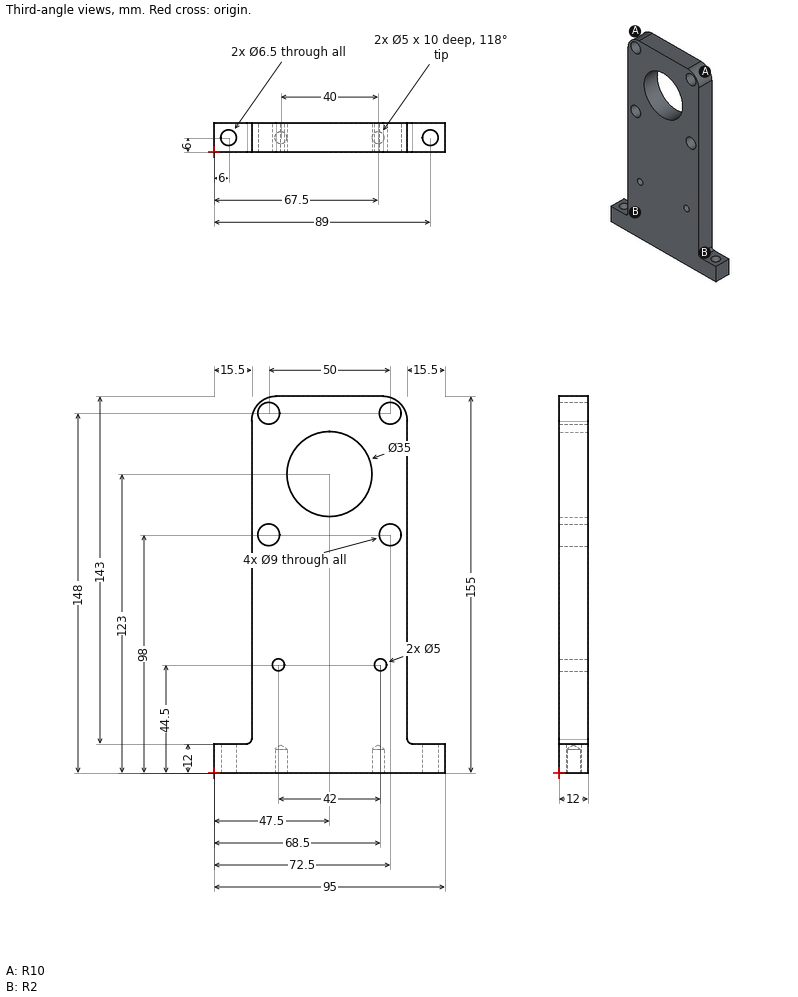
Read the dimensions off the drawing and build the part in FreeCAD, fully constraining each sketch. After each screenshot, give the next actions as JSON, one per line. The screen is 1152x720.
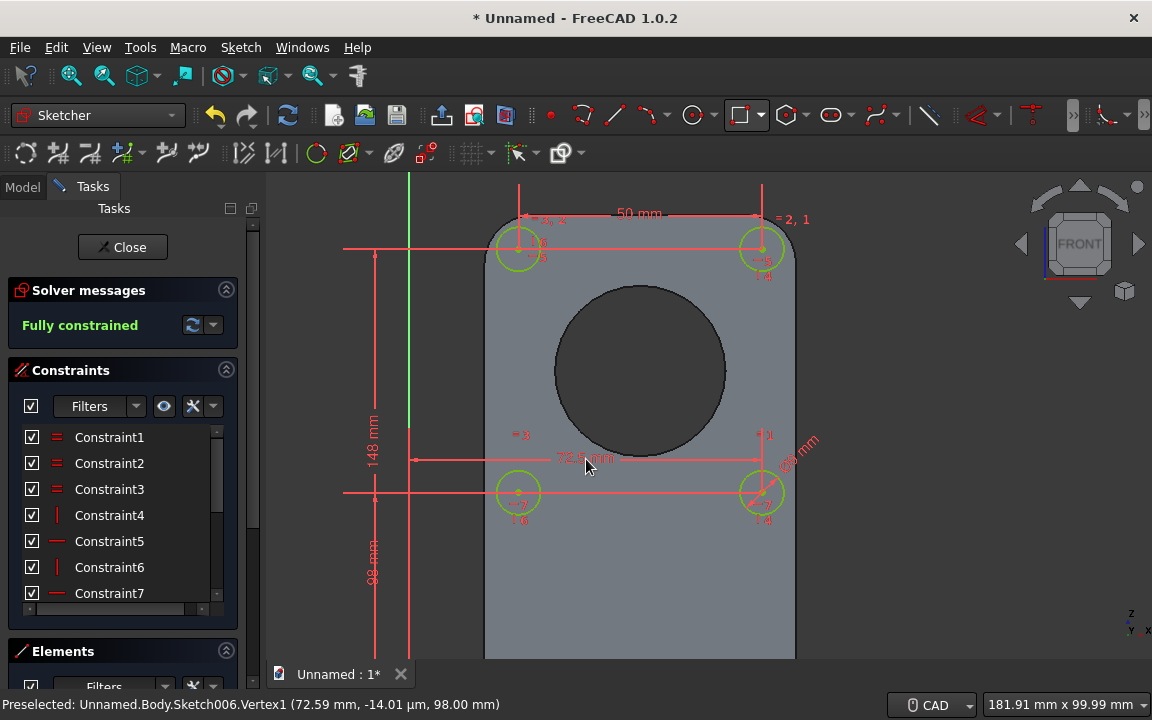
{"action": "left_click", "coordinate": [123, 247]}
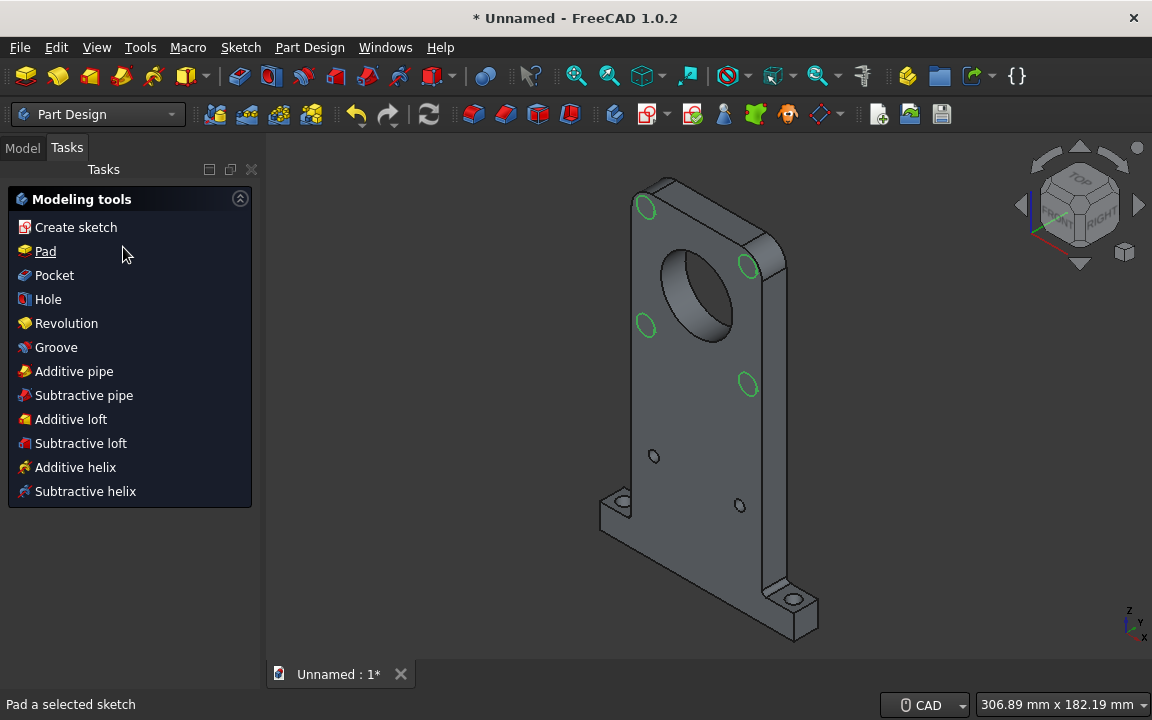
{"action": "left_click", "coordinate": [272, 76]}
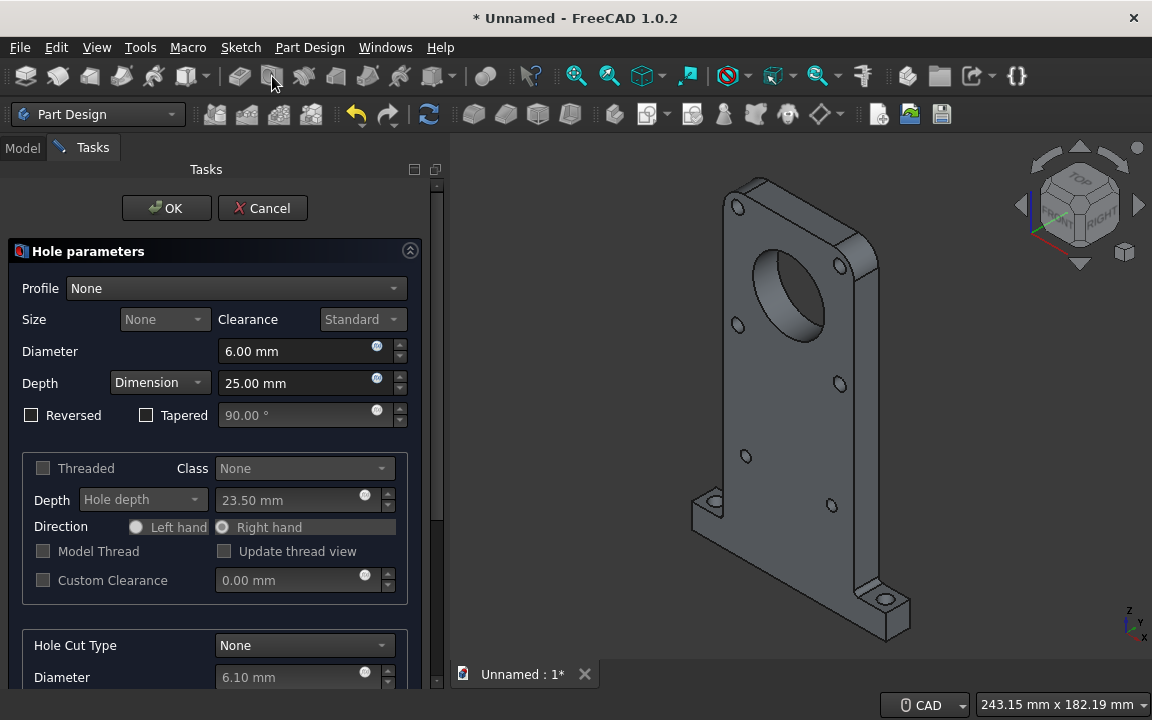
{"action": "triple_click", "coordinate": [305, 351]}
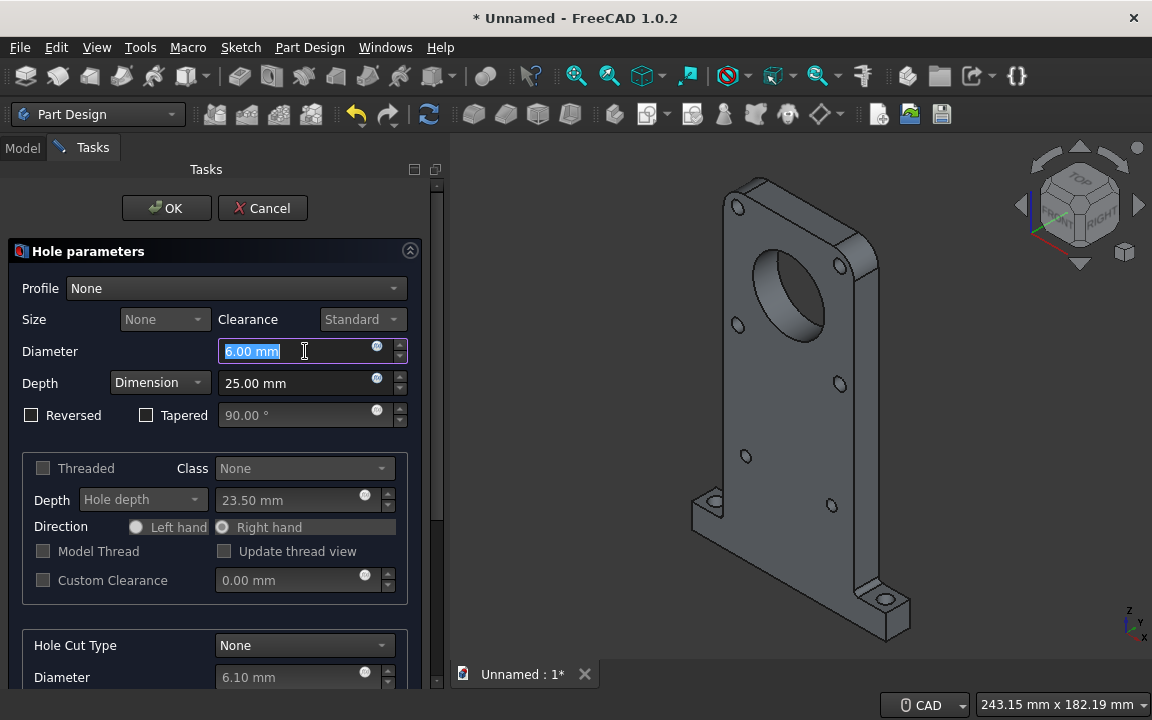
{"action": "type", "text": "9"}
{"action": "key", "text": "Tab"}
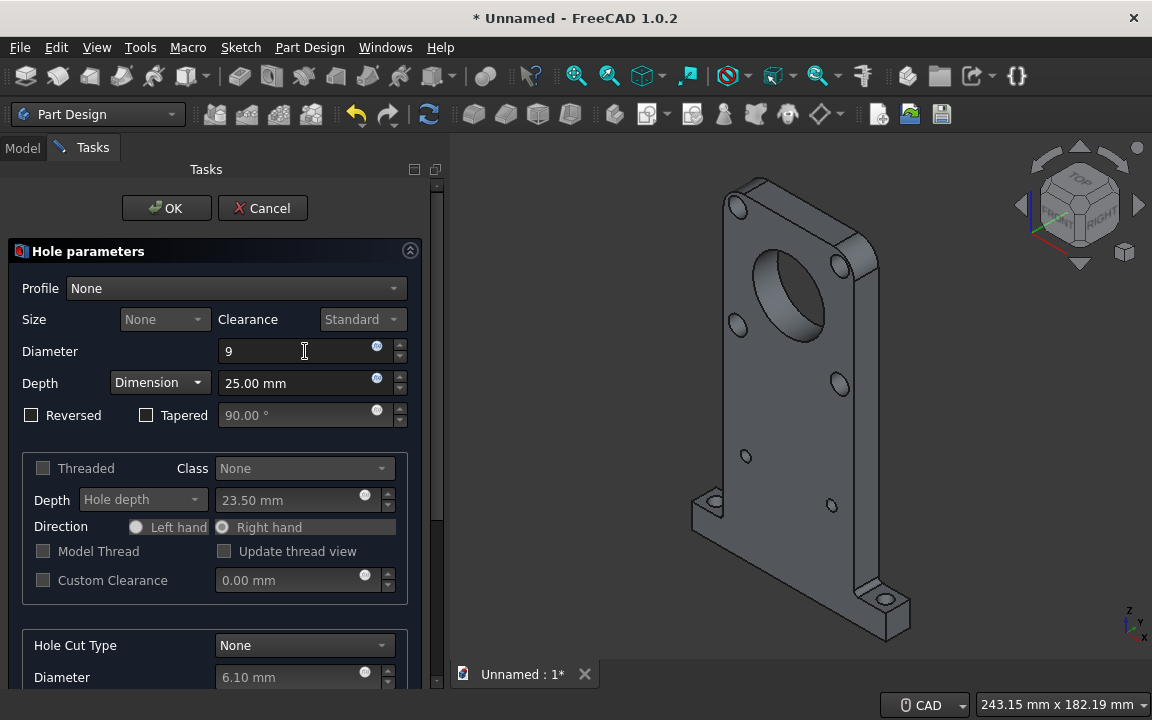
{"action": "left_click", "coordinate": [161, 382]}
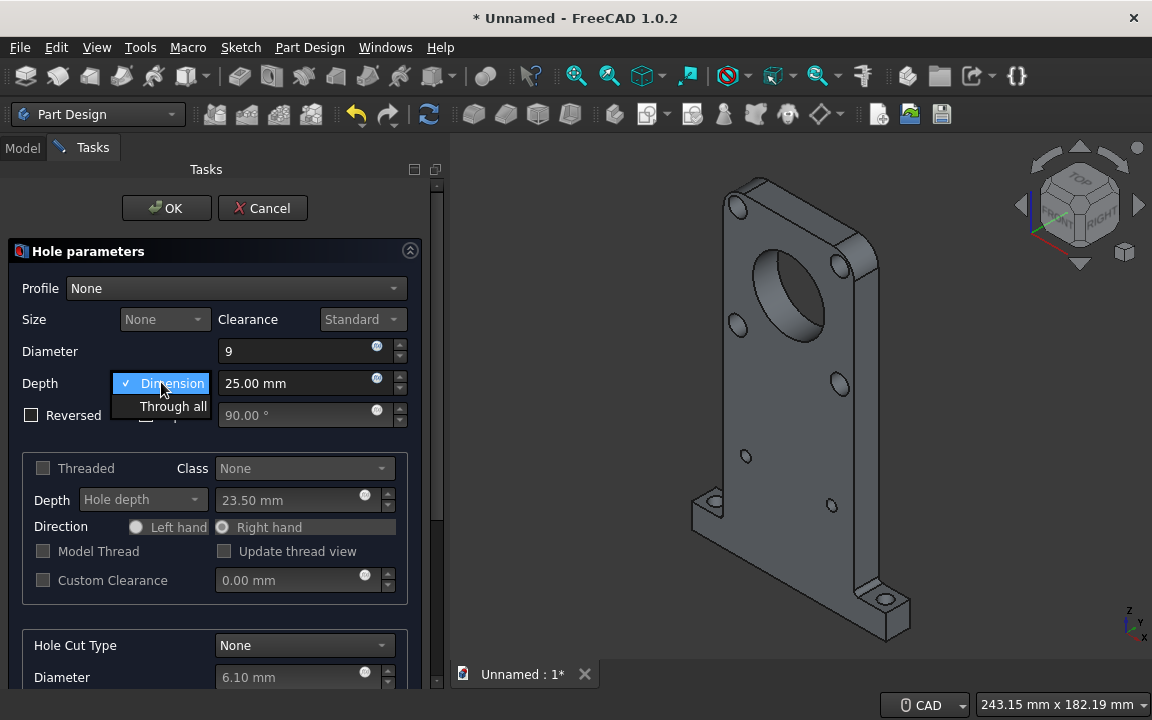
{"action": "left_click", "coordinate": [160, 406]}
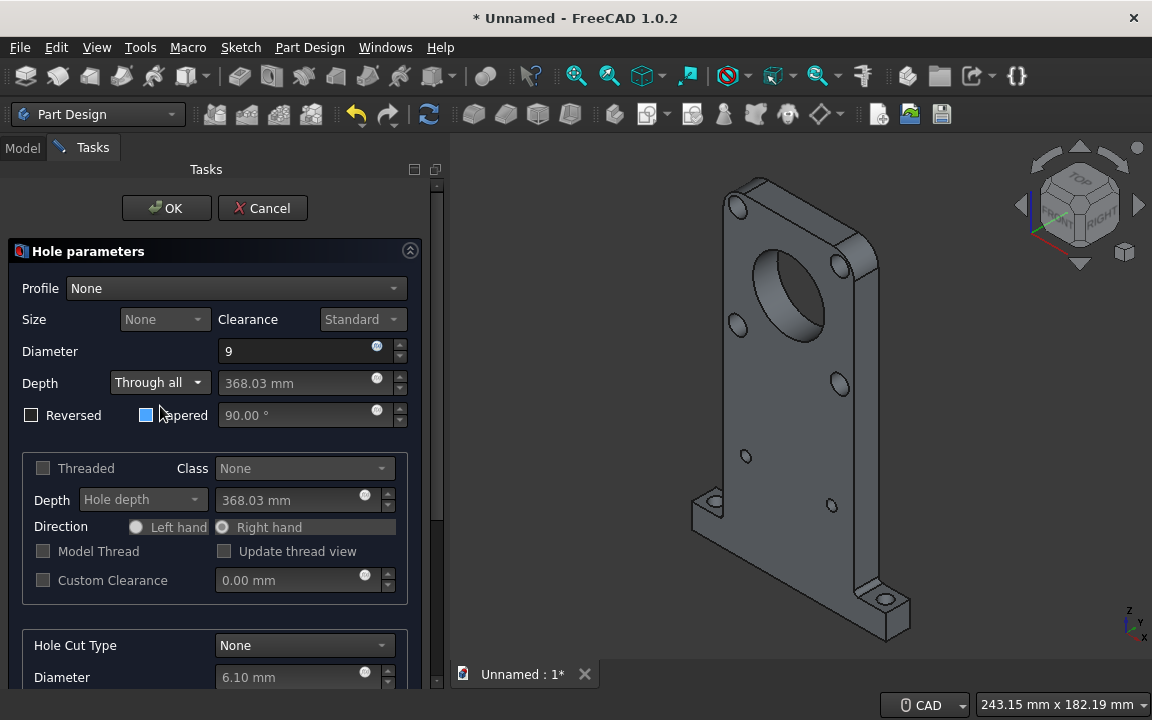
{"action": "left_click", "coordinate": [167, 208]}